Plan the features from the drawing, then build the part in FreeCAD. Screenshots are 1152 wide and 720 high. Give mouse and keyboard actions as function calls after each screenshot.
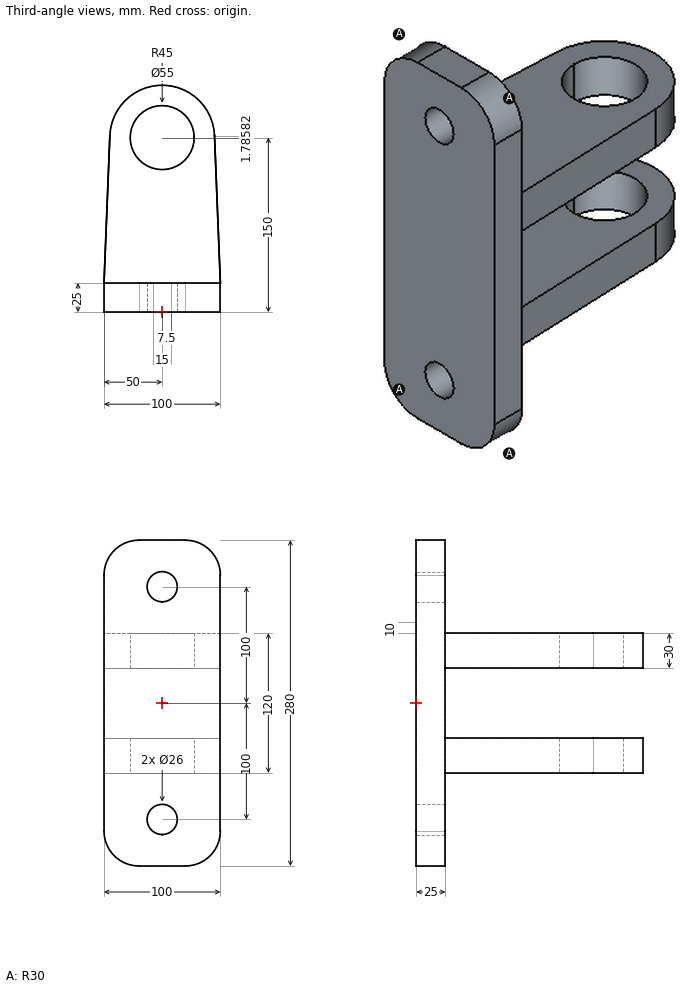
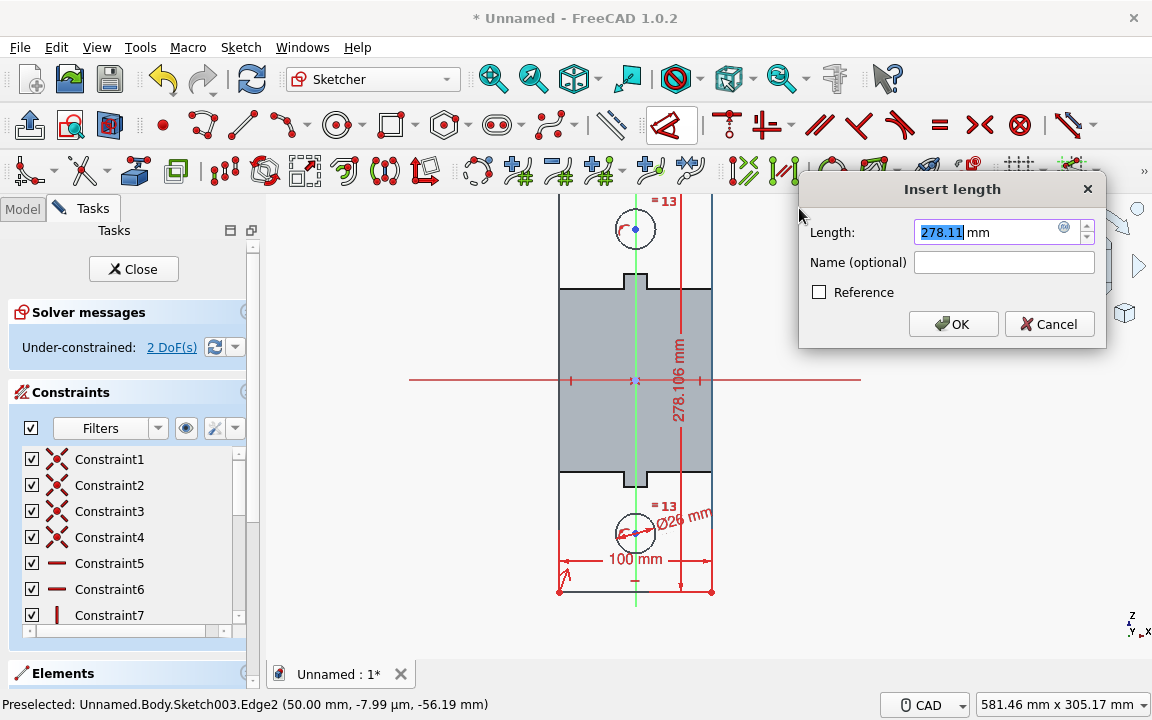
text(280)
key(Return)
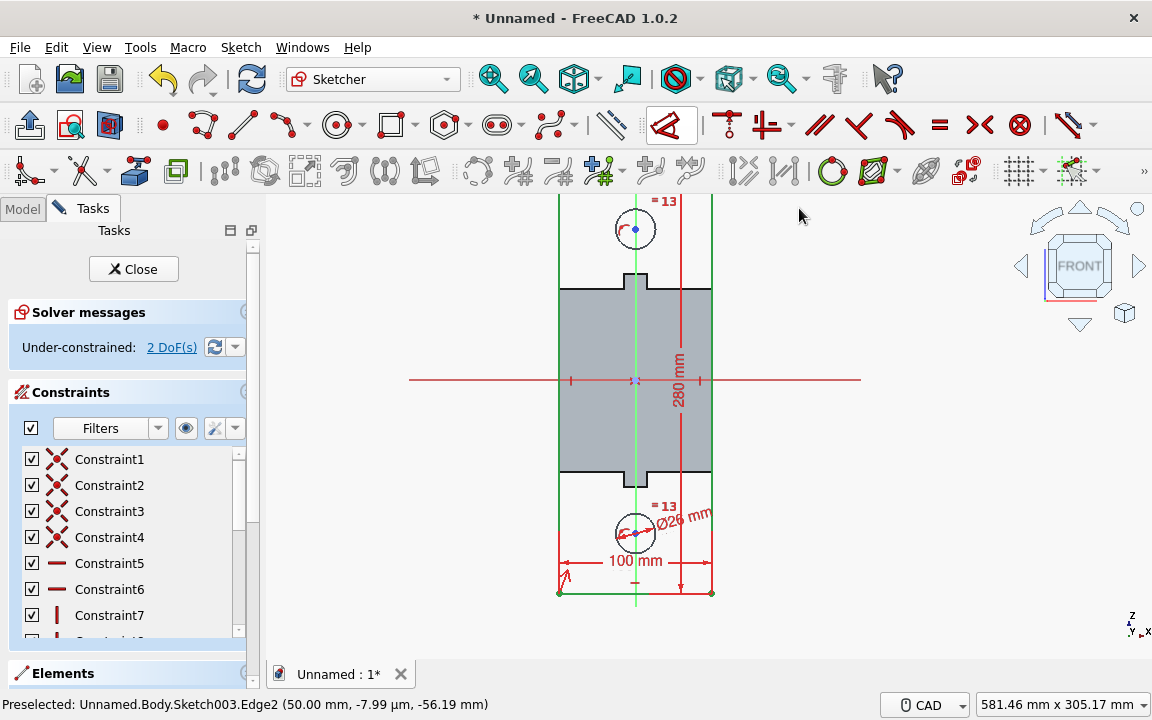
click(636, 534)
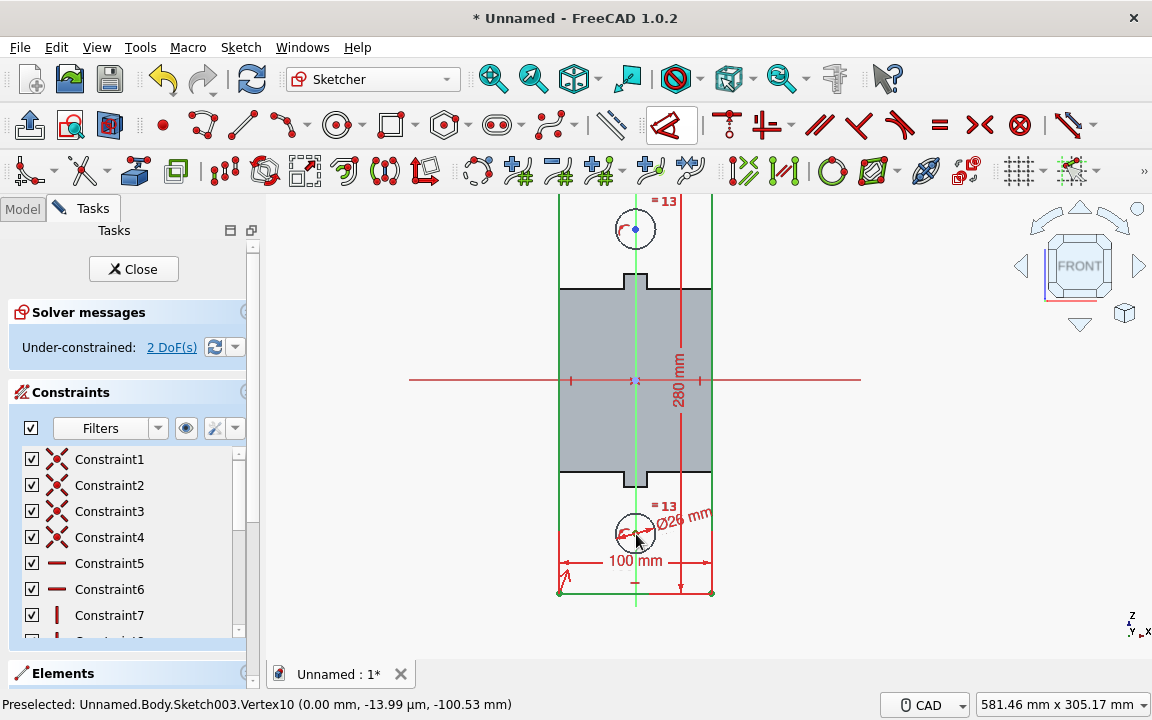
click(692, 126)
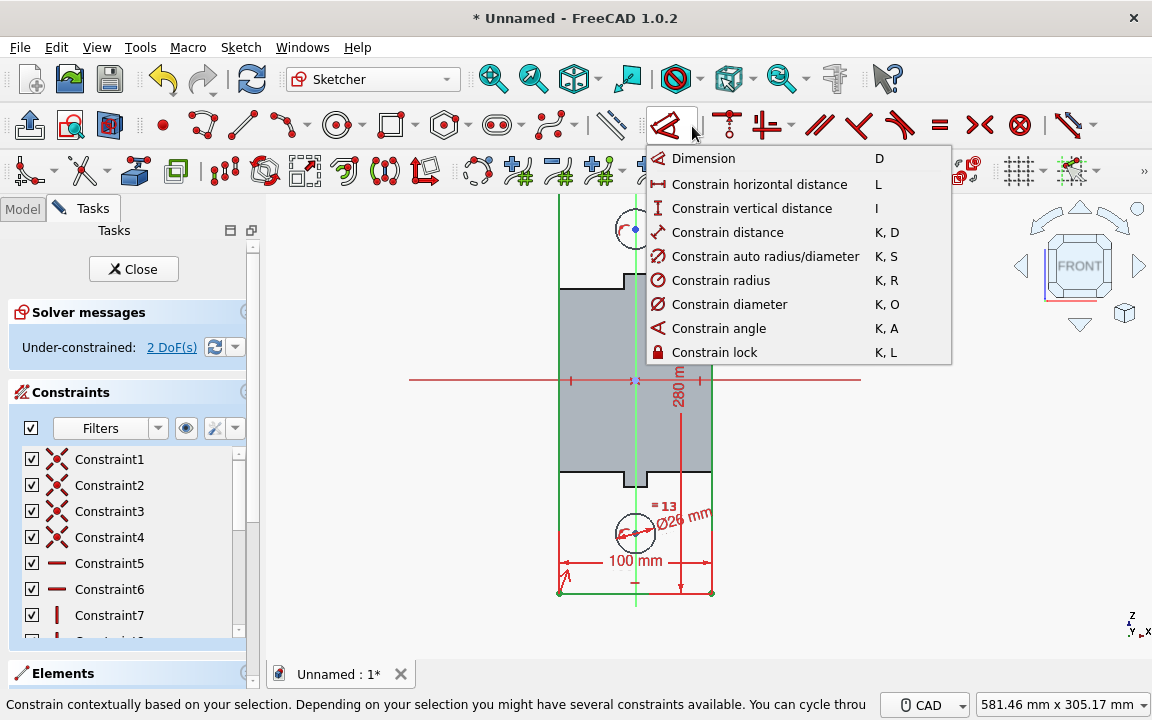
click(799, 208)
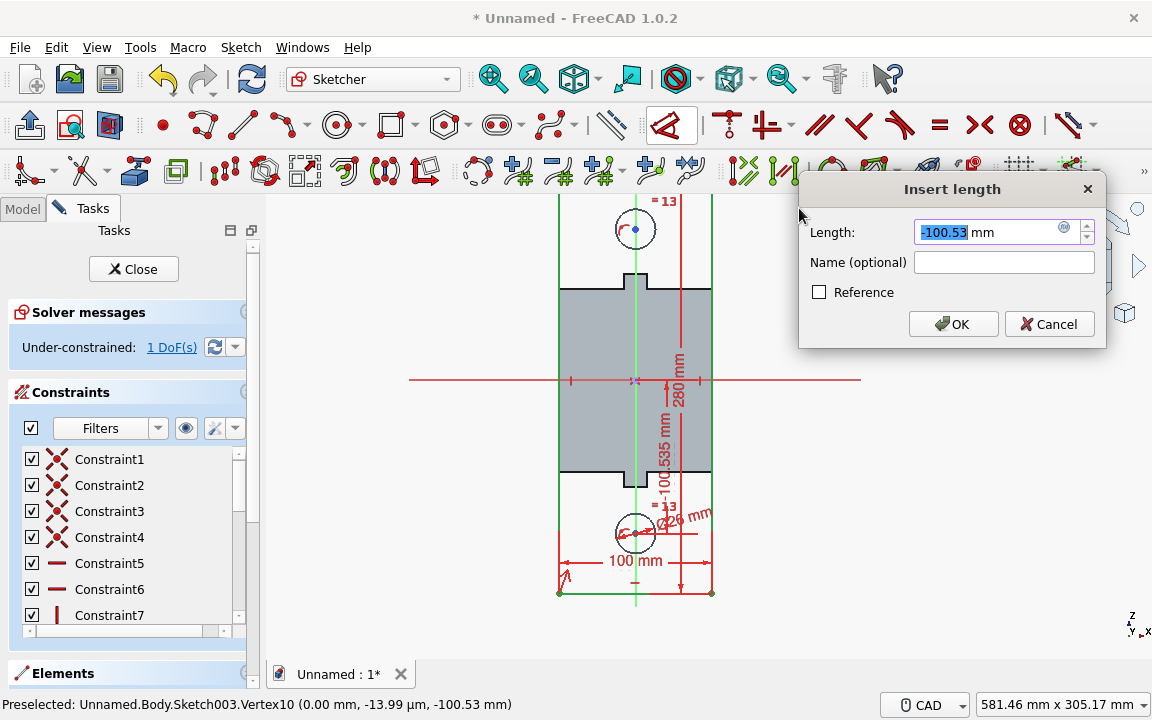
text(-100)
key(Return)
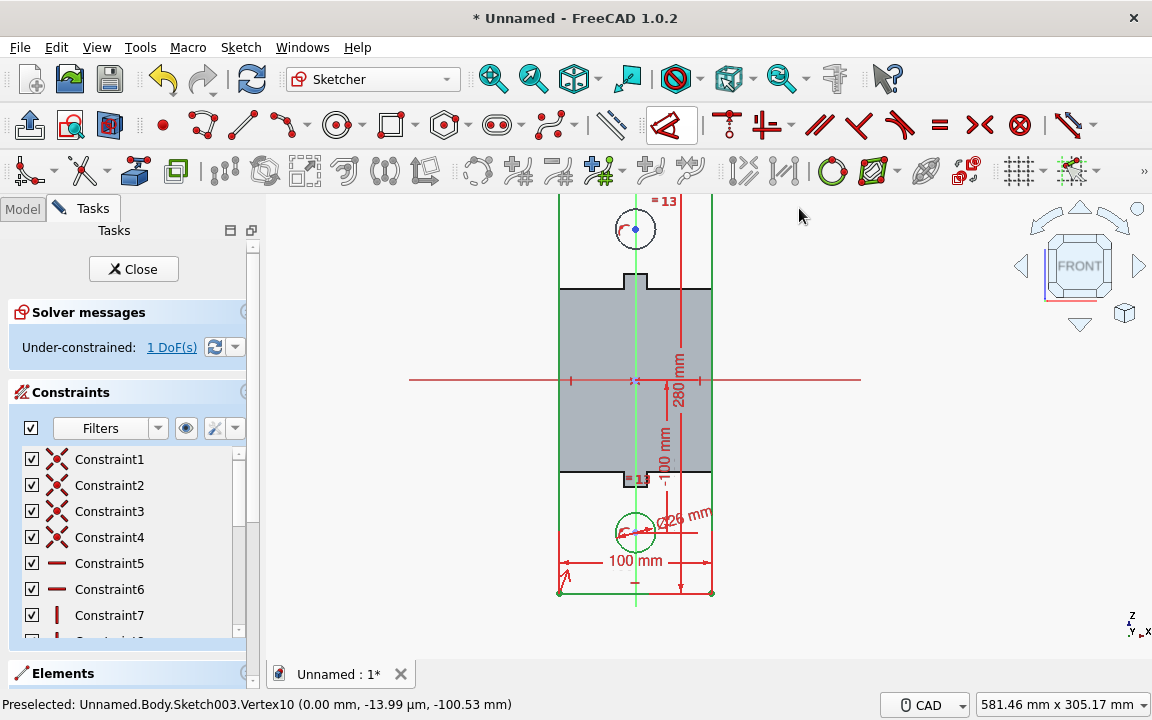
click(636, 229)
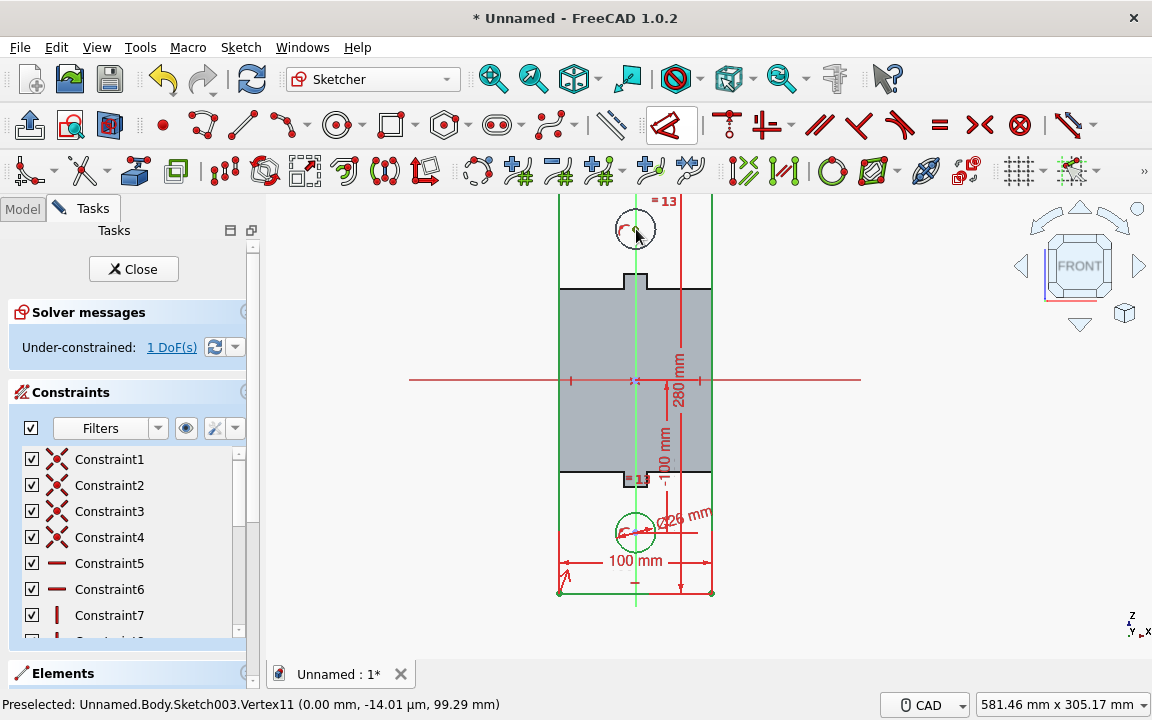
click(692, 126)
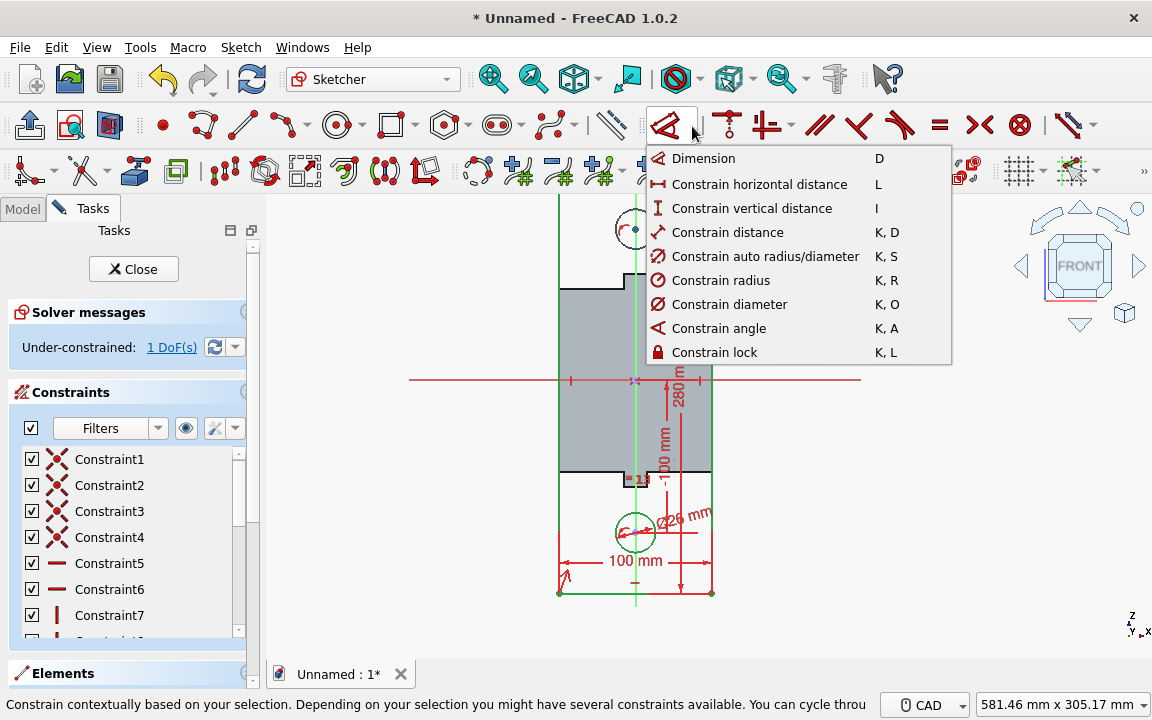
click(799, 208)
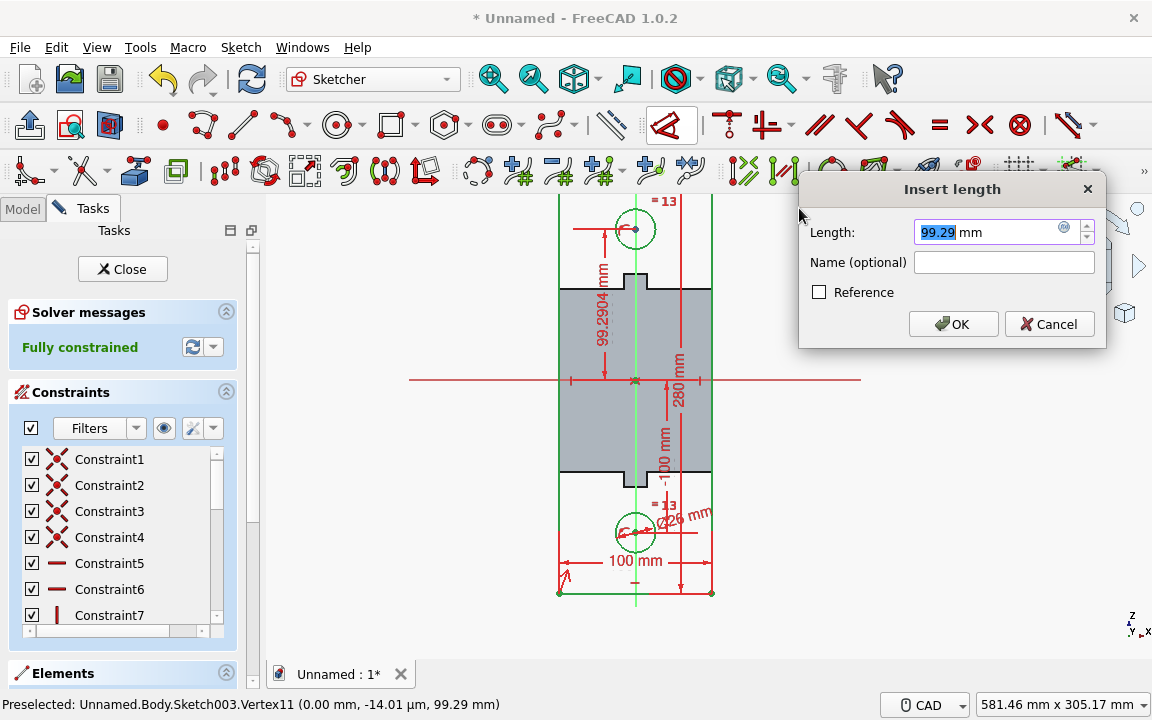
text(100)
key(Return)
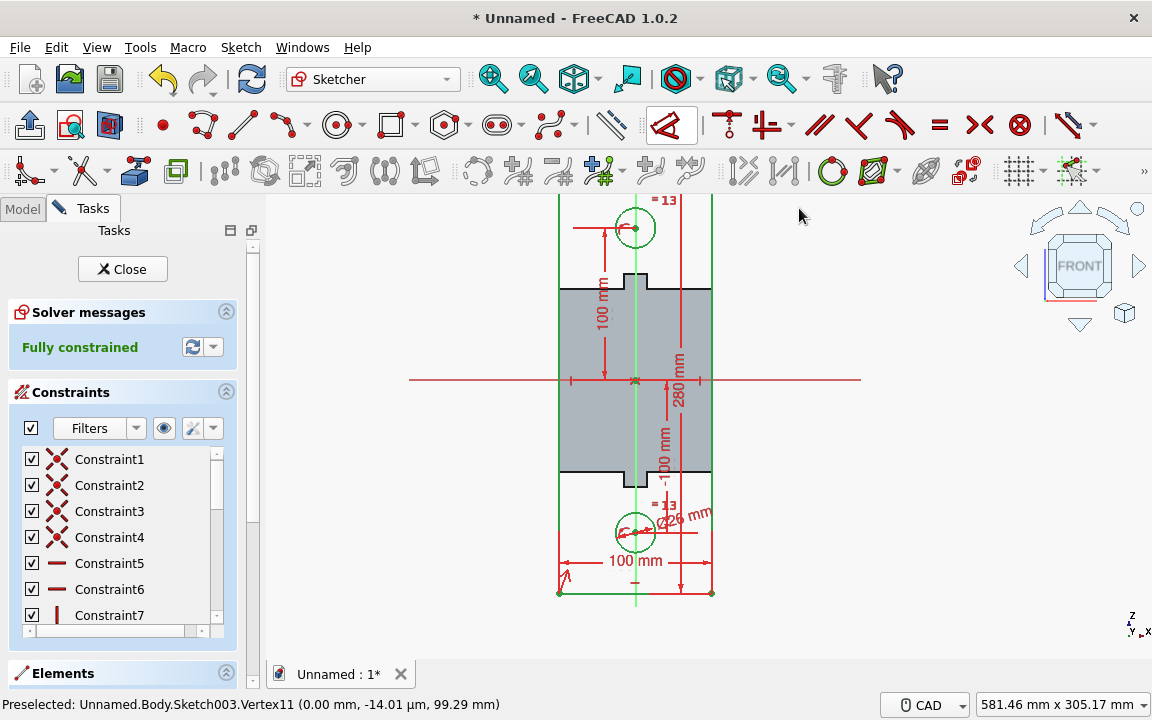
click(123, 269)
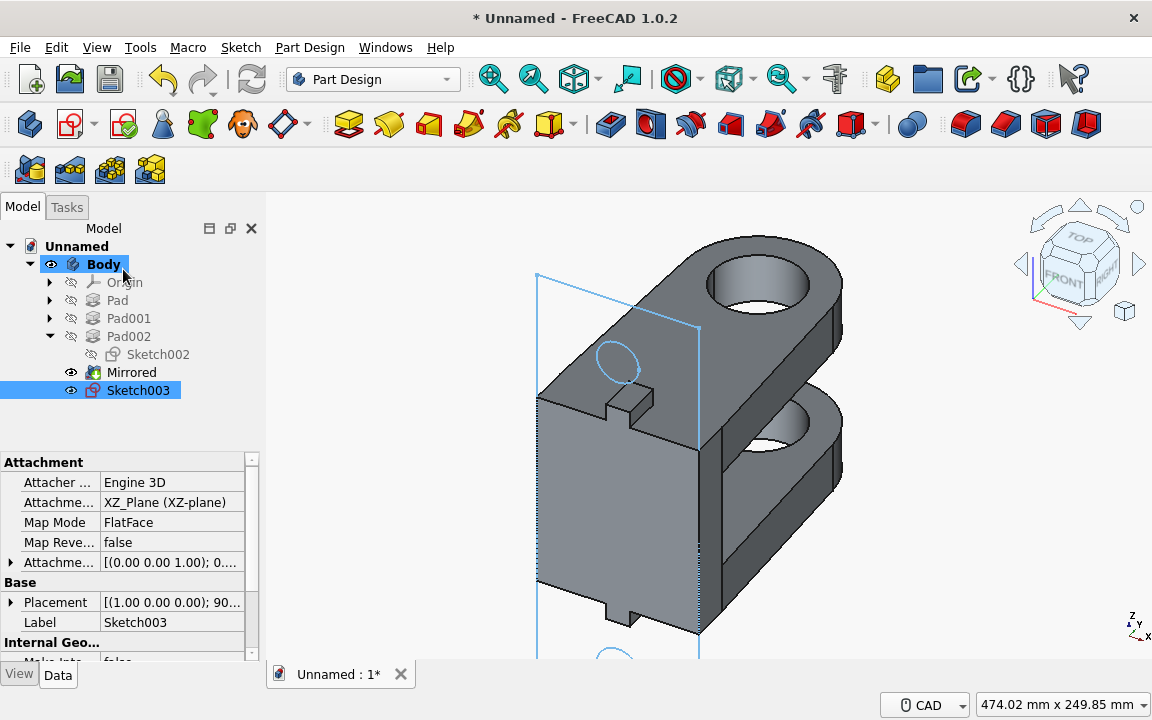
click(350, 124)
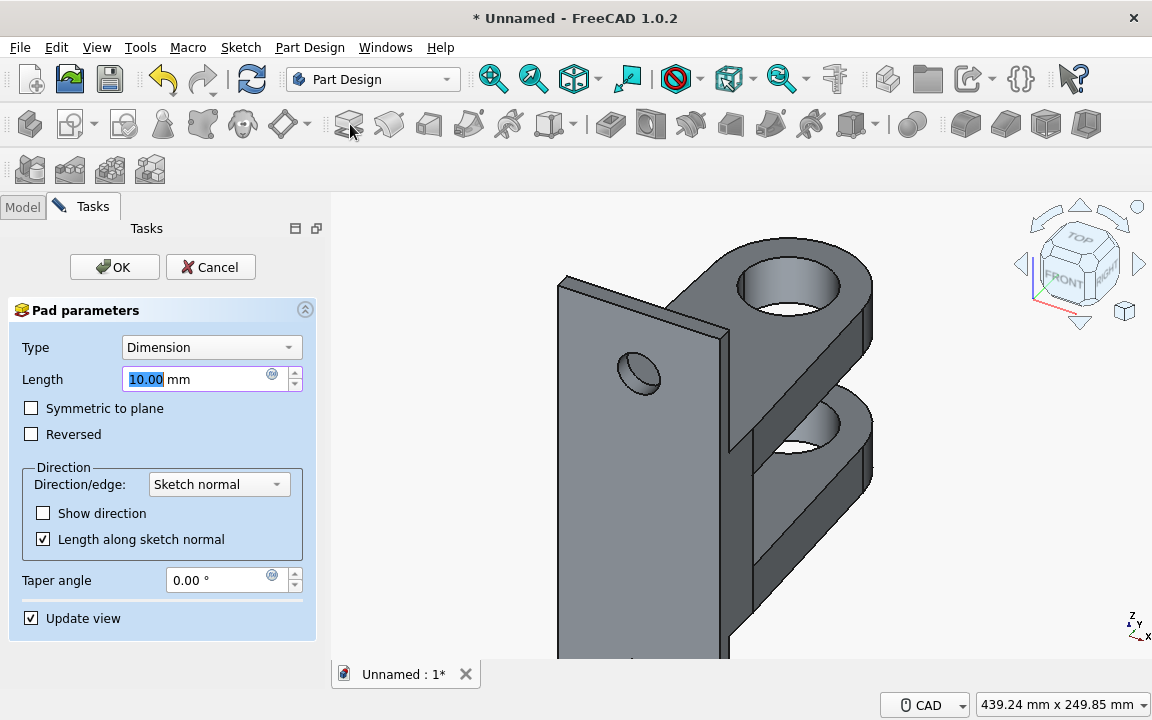
text(25)
key(Tab)